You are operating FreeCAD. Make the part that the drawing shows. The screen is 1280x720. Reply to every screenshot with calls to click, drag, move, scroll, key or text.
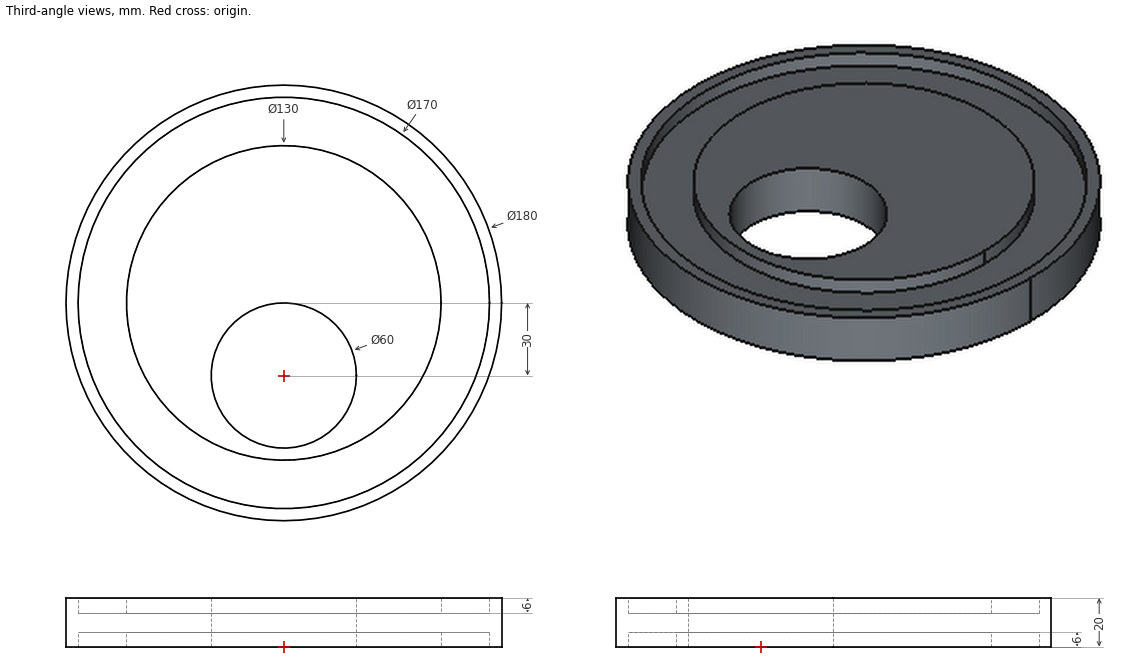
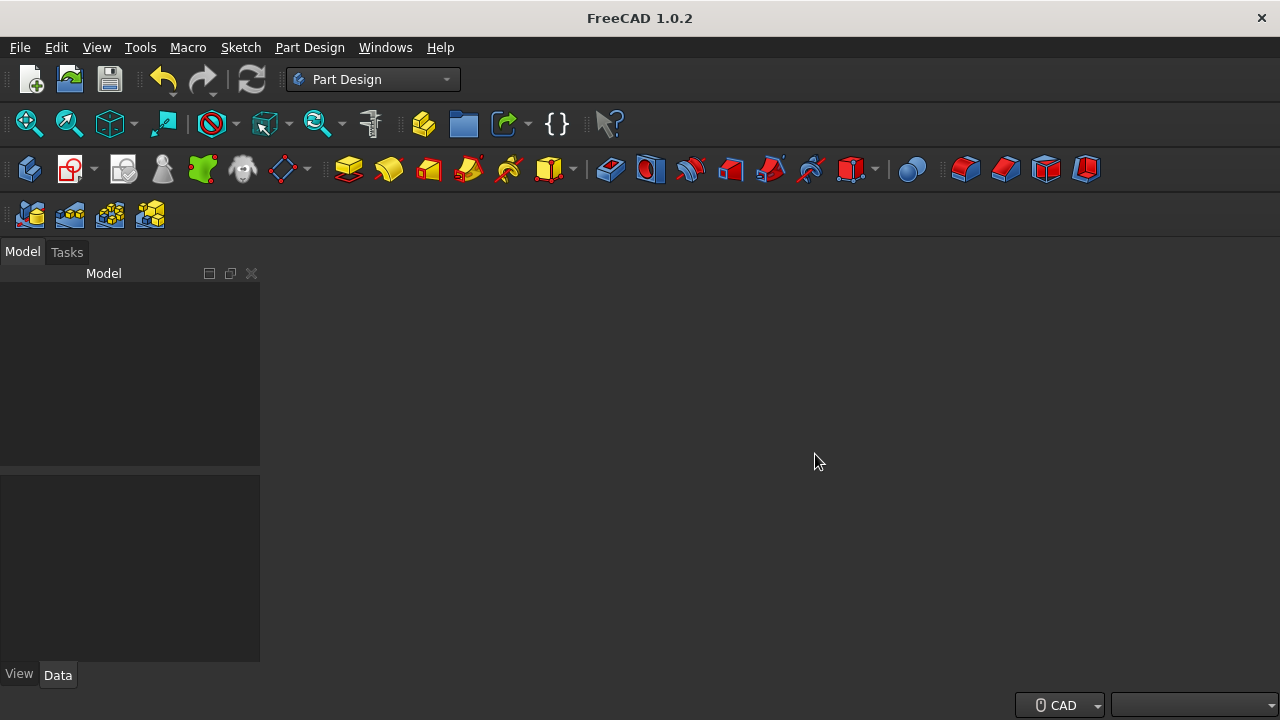
click(30, 80)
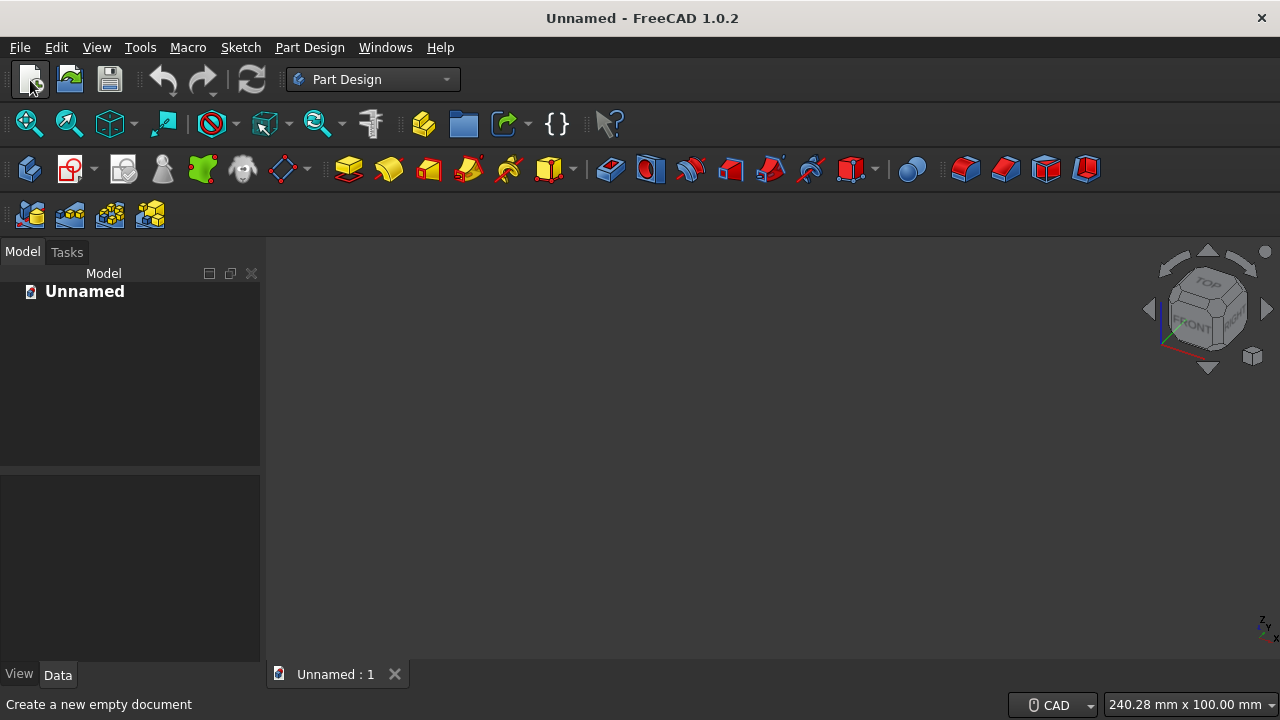
click(70, 170)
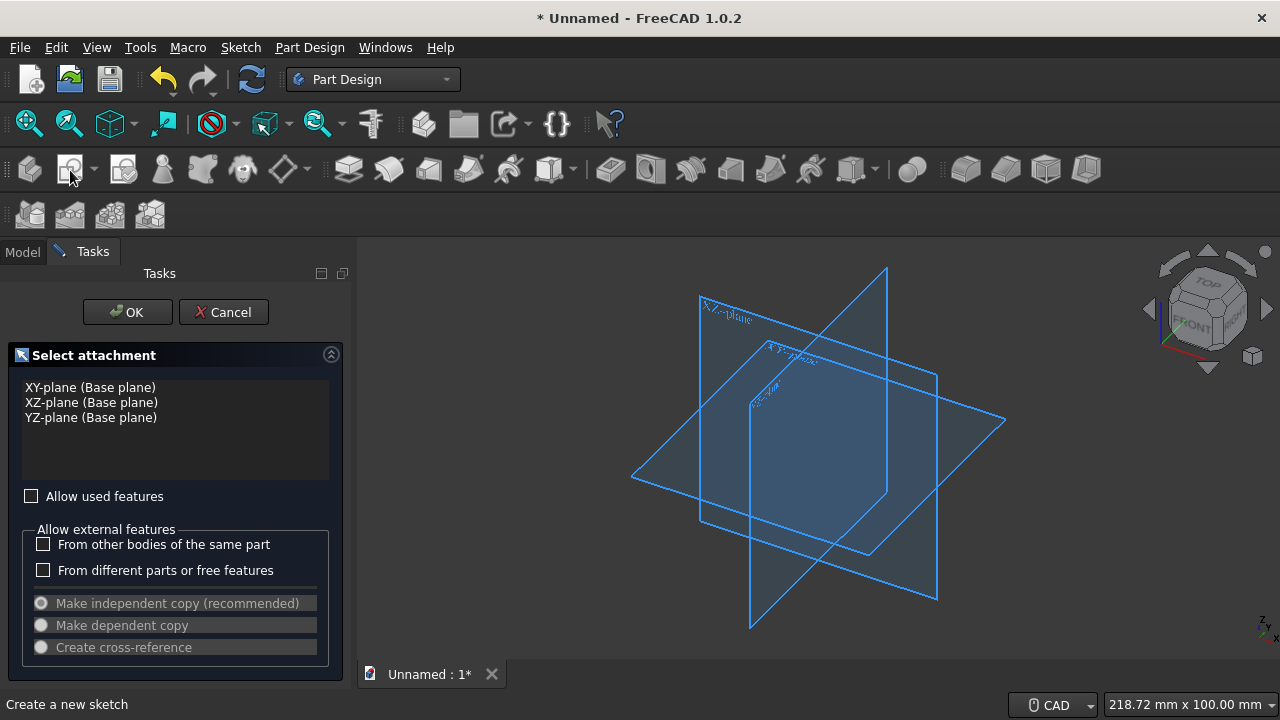
click(82, 388)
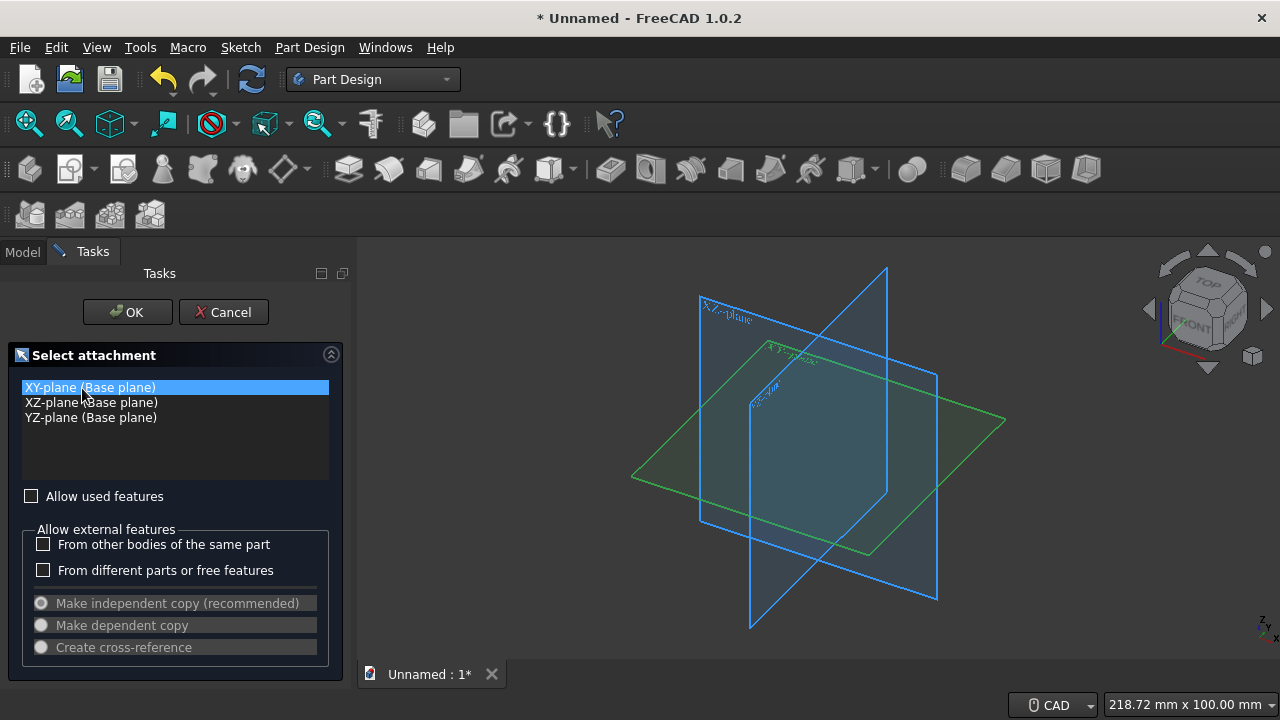
click(128, 312)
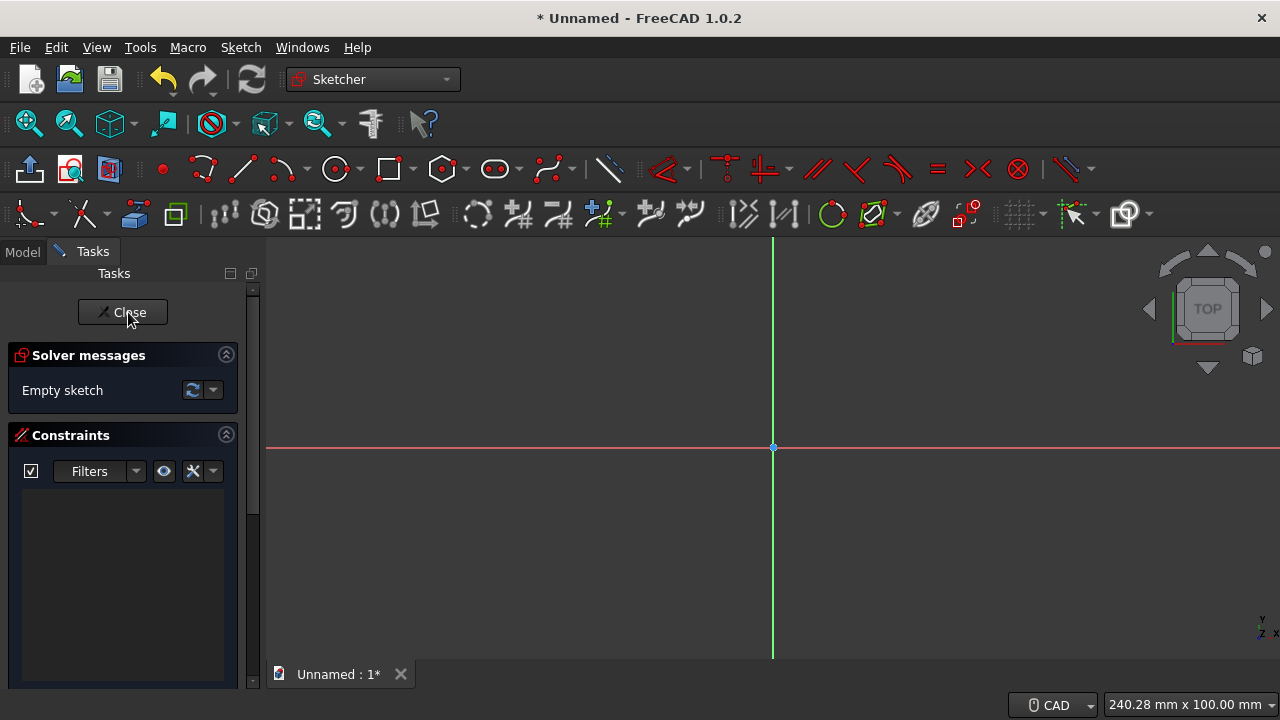
scroll(665, 522, down, 5)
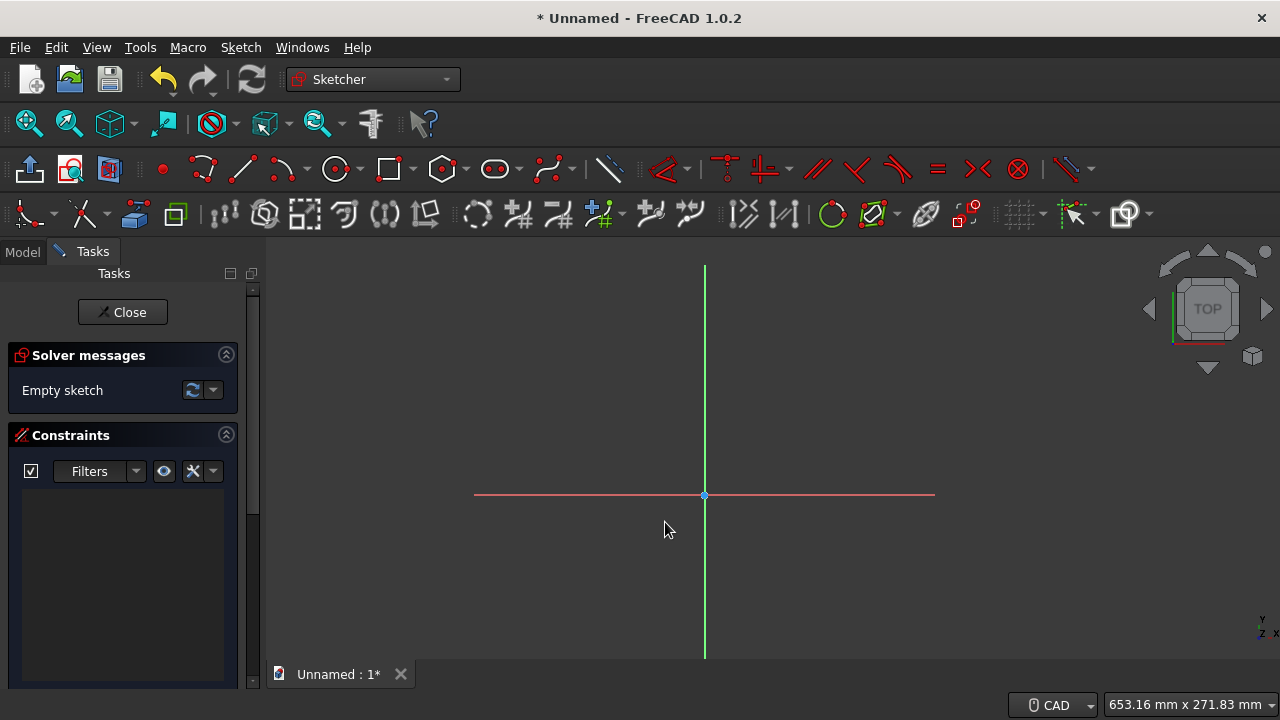
click(336, 170)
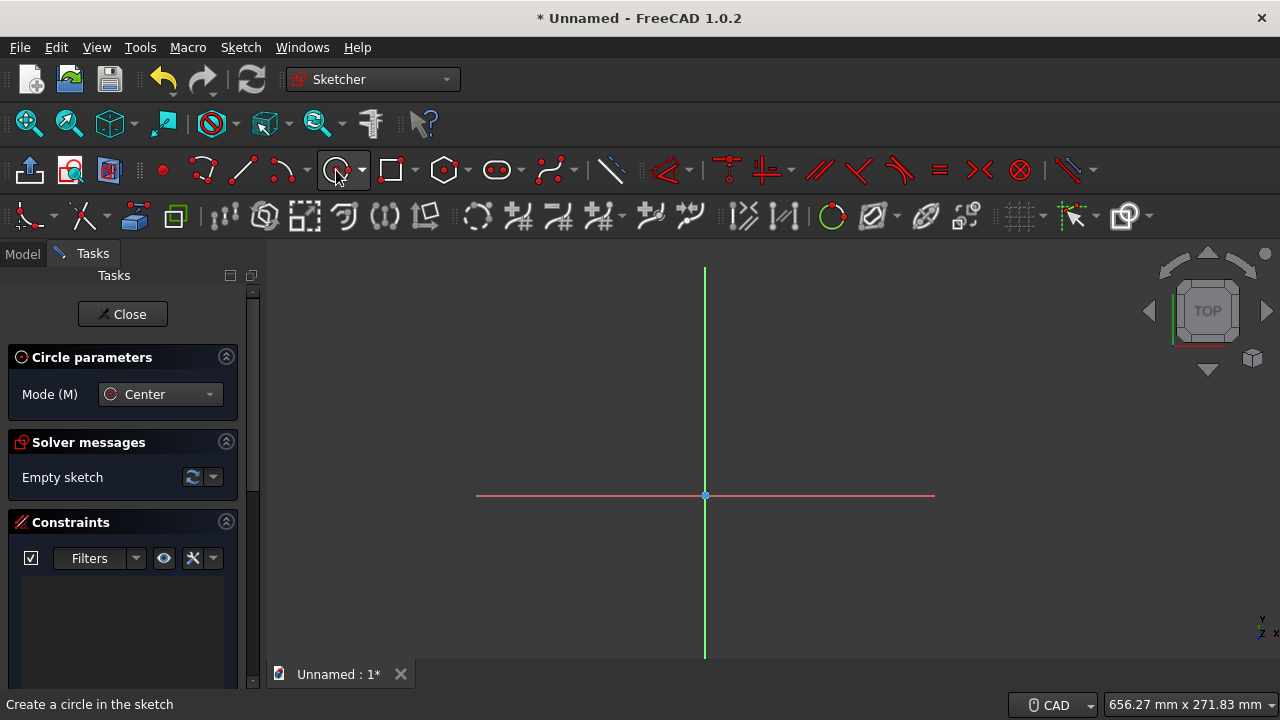
click(705, 450)
move(804, 351)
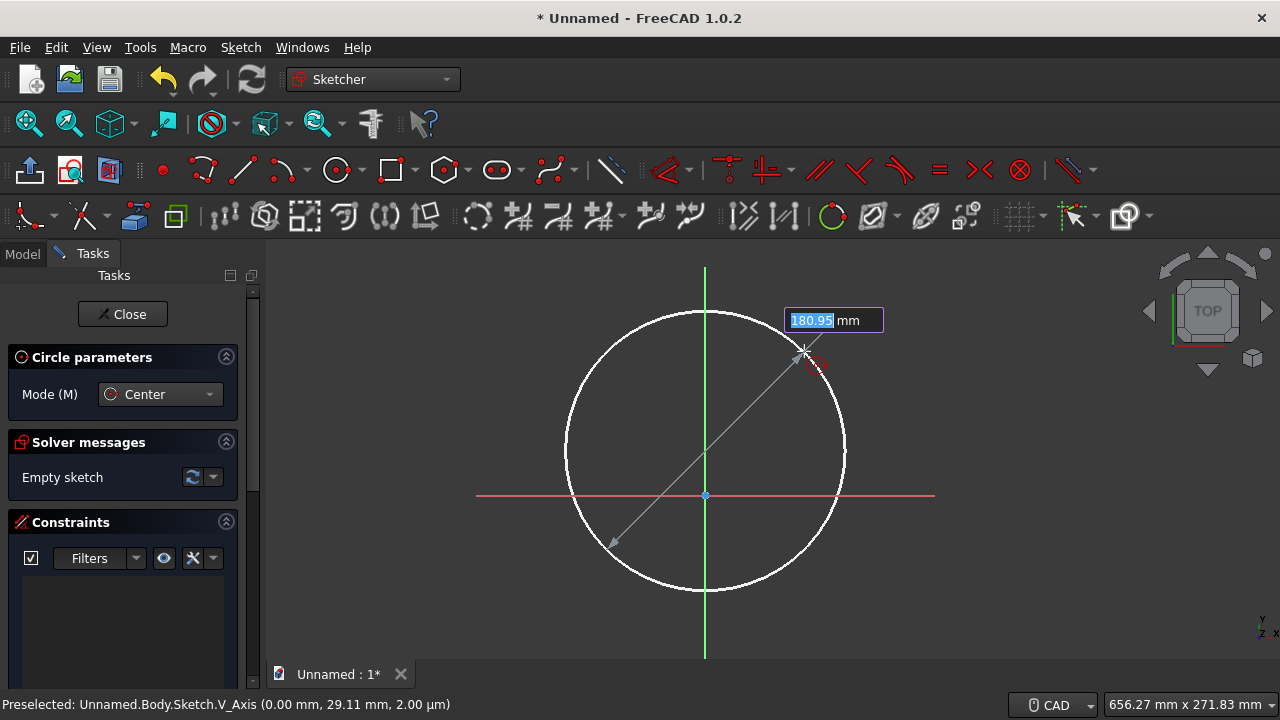
text(180)
key(Return)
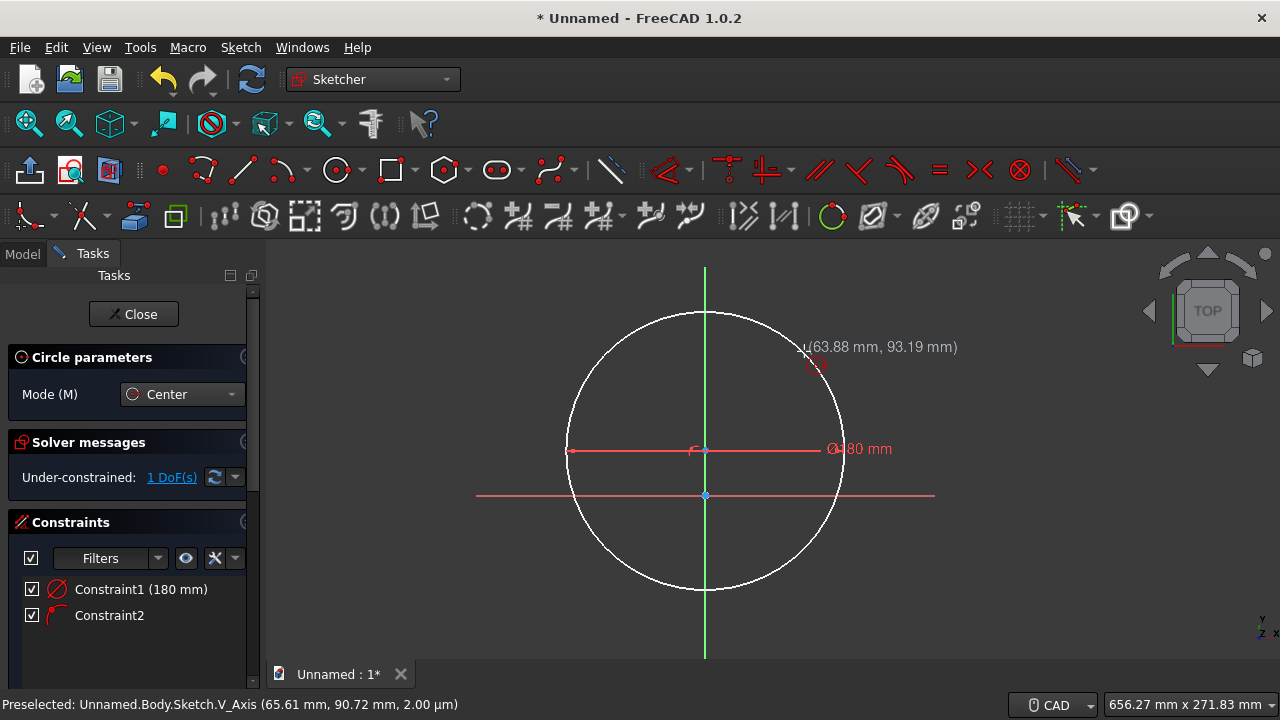
click(705, 496)
move(738, 463)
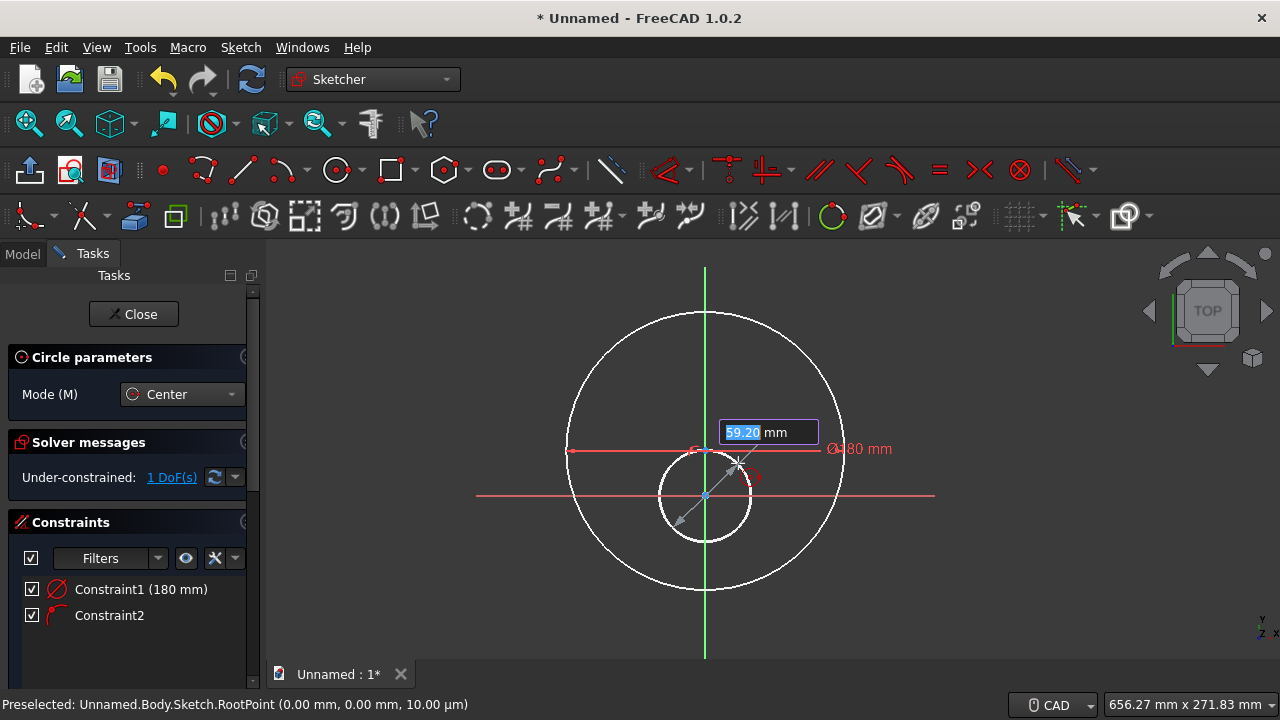
text(60)
key(Return)
key(Escape)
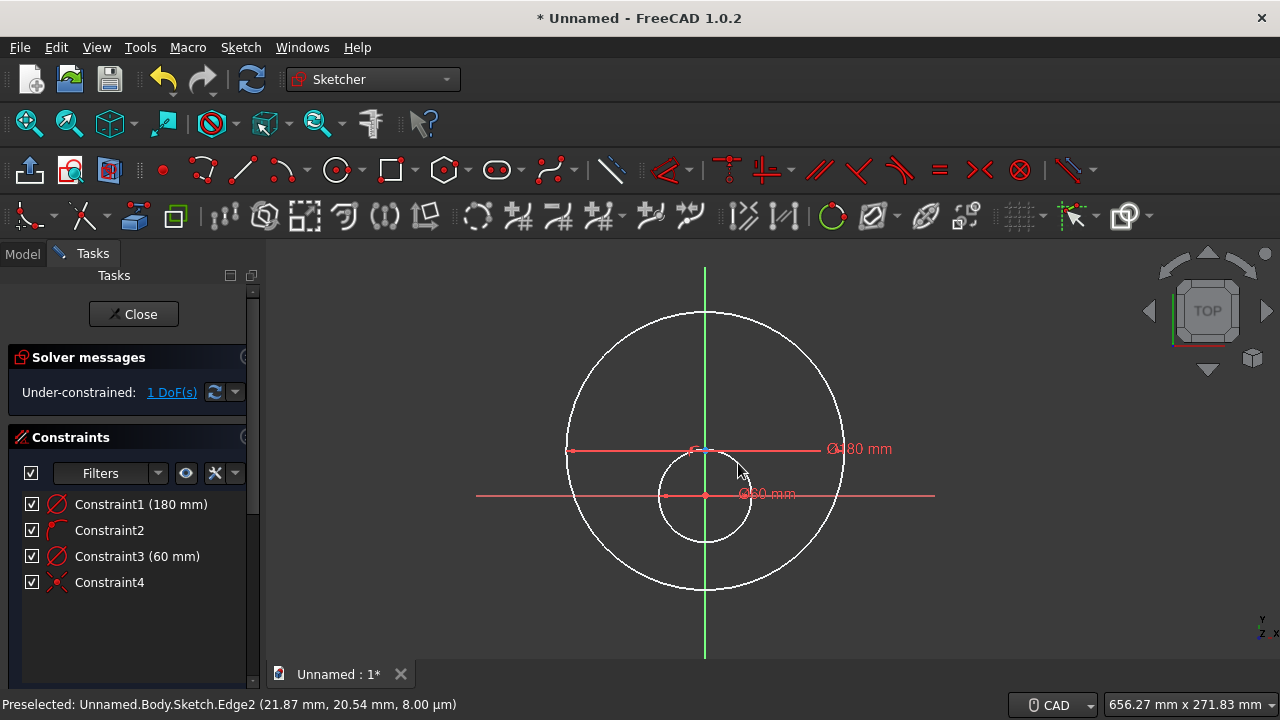
click(705, 451)